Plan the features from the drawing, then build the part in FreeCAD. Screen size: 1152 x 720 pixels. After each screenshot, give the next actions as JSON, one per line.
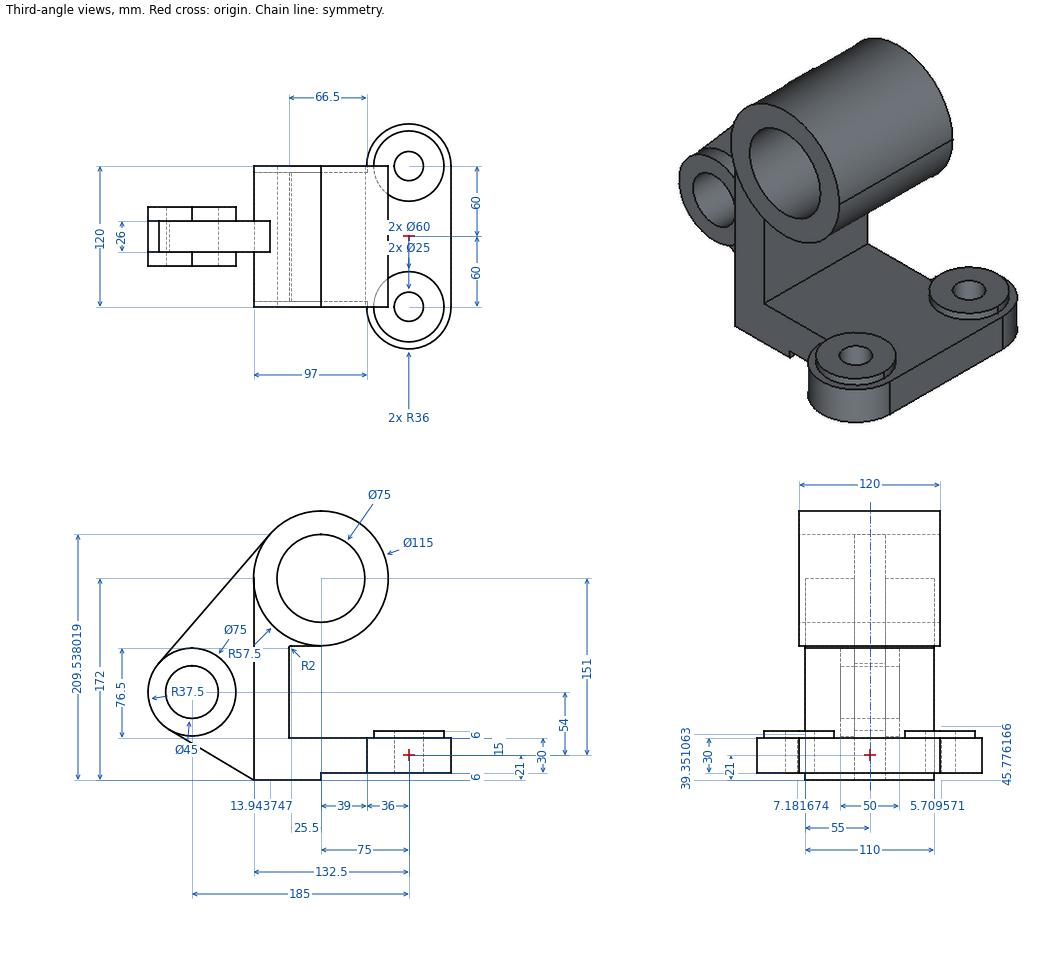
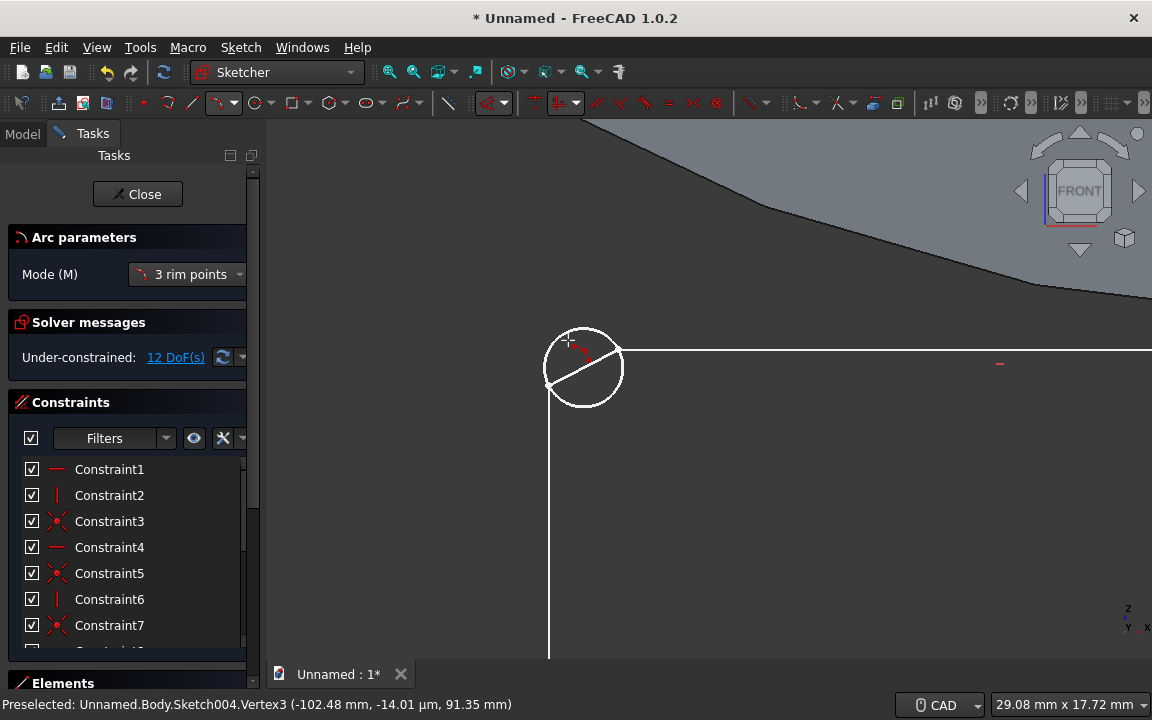
{"action": "left_click", "coordinate": [566, 338]}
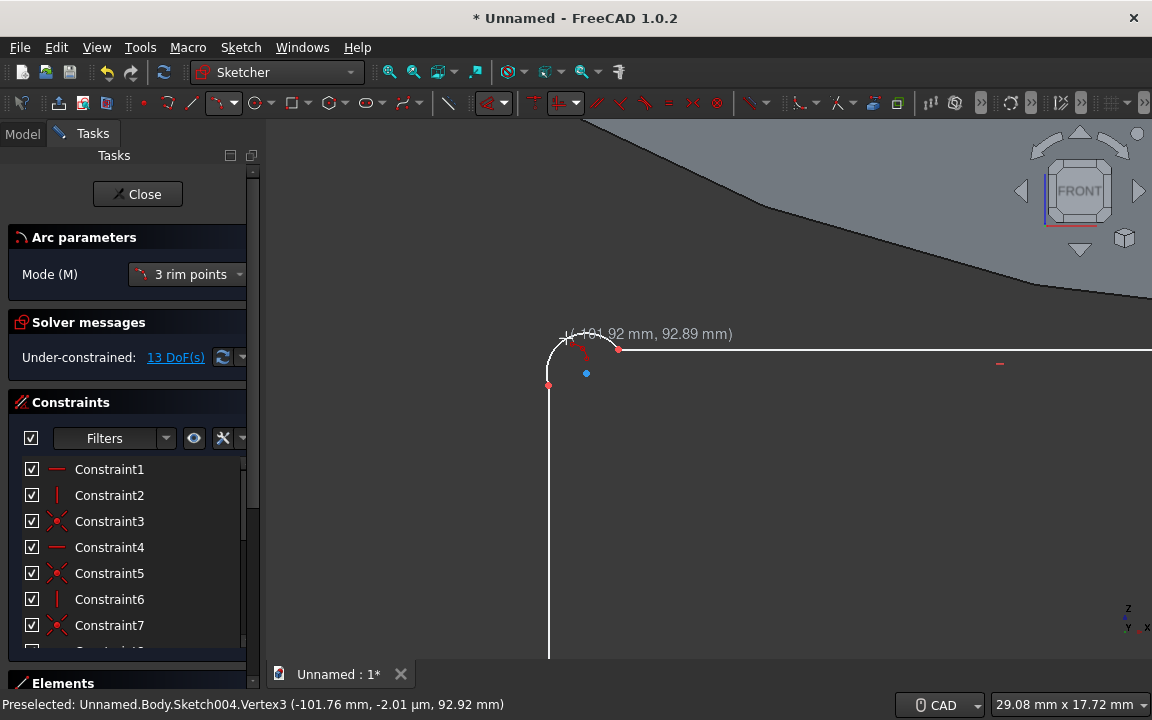
{"action": "scroll", "coordinate": [575, 337], "scroll_direction": "down", "scroll_amount": 14}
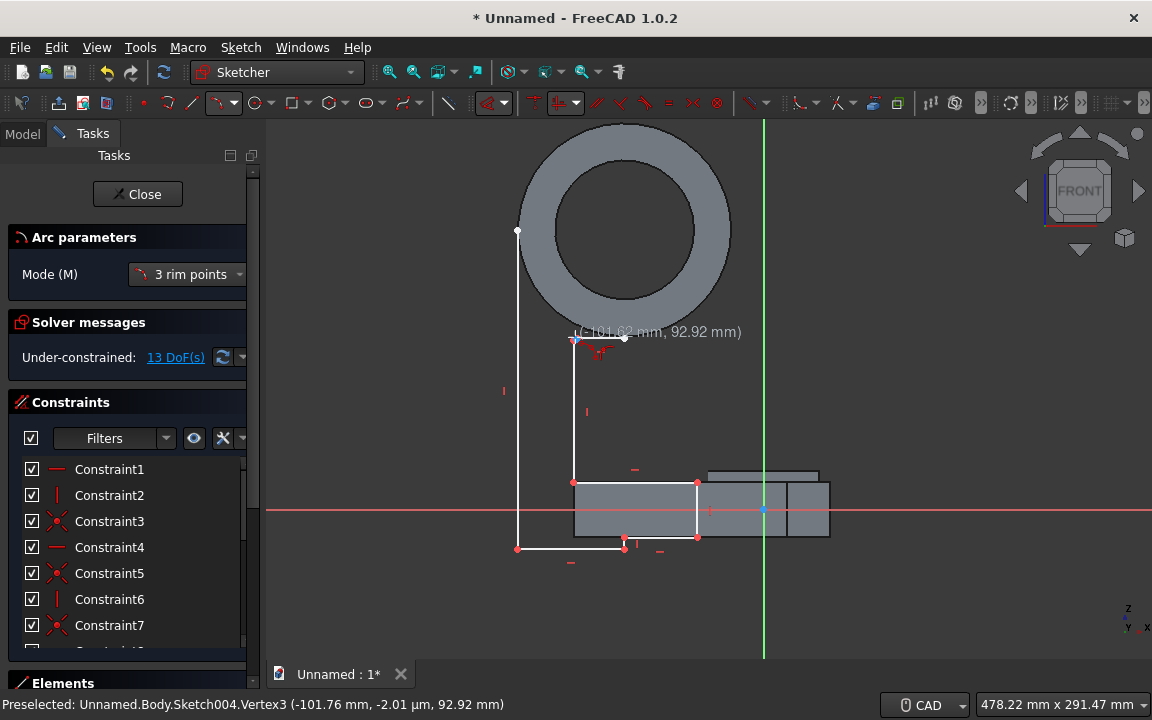
{"action": "left_click", "coordinate": [518, 231]}
{"action": "left_click", "coordinate": [624, 338]}
{"action": "left_click", "coordinate": [549, 305]}
{"action": "key", "text": "Escape"}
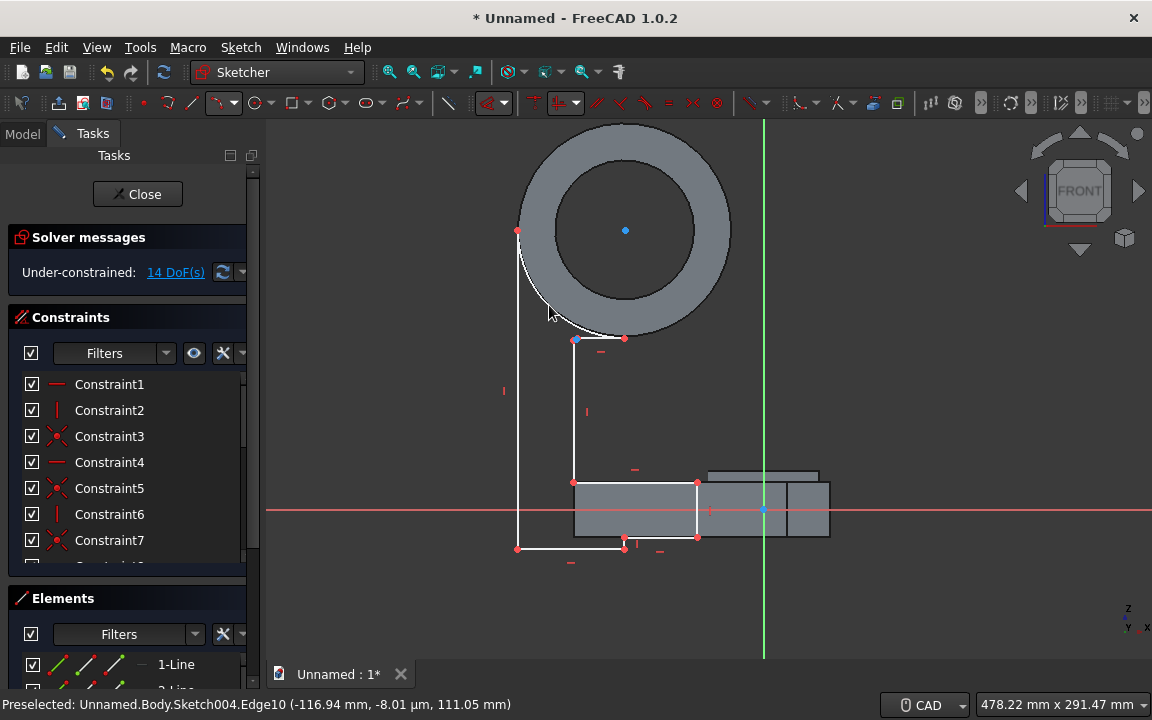
{"action": "scroll", "coordinate": [587, 338], "scroll_direction": "up", "scroll_amount": 4}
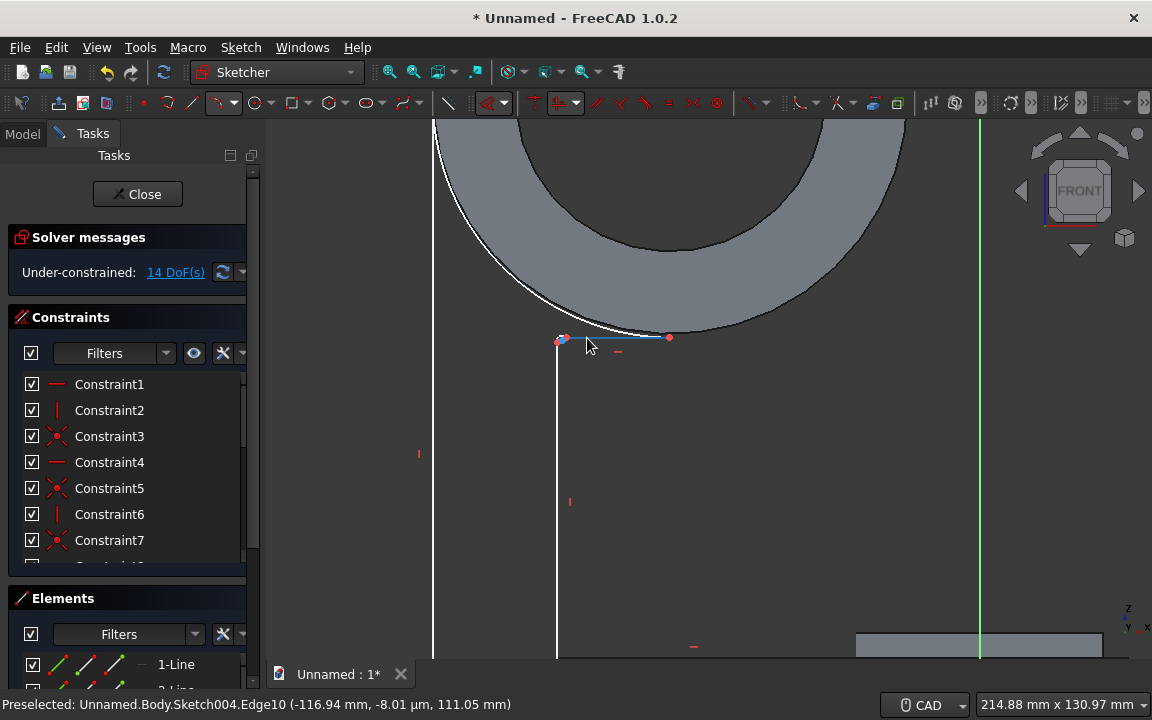
{"action": "left_click", "coordinate": [587, 338]}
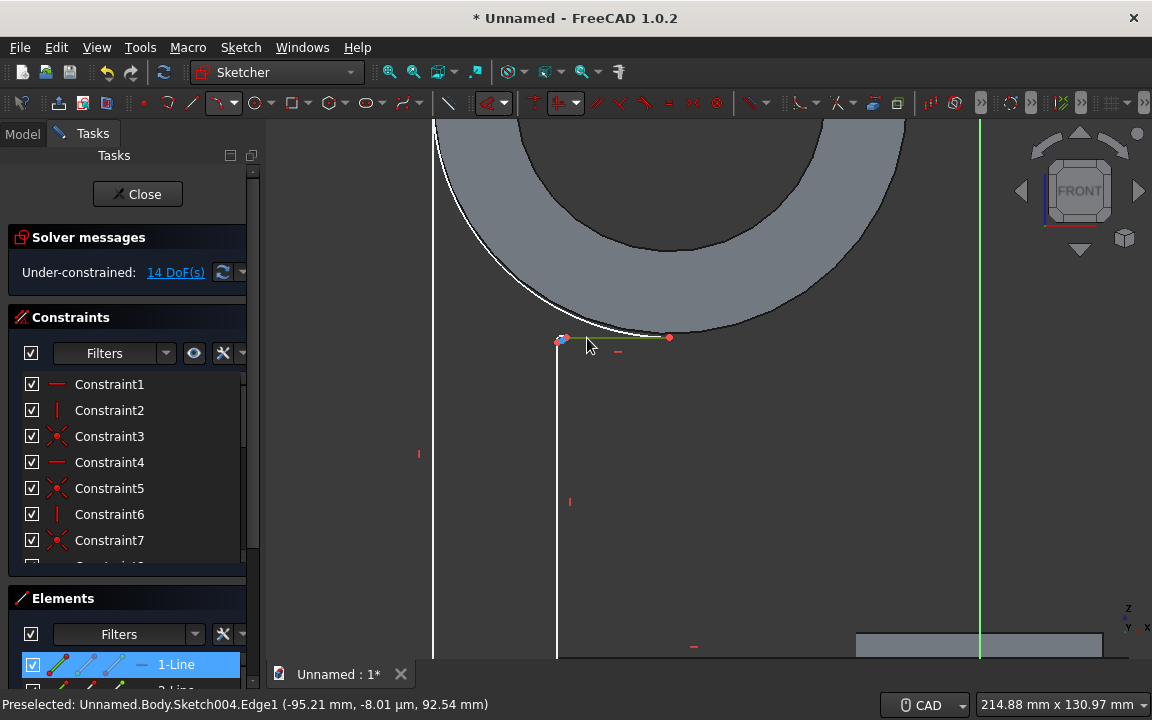
{"action": "scroll", "coordinate": [560, 336], "scroll_direction": "up", "scroll_amount": 5}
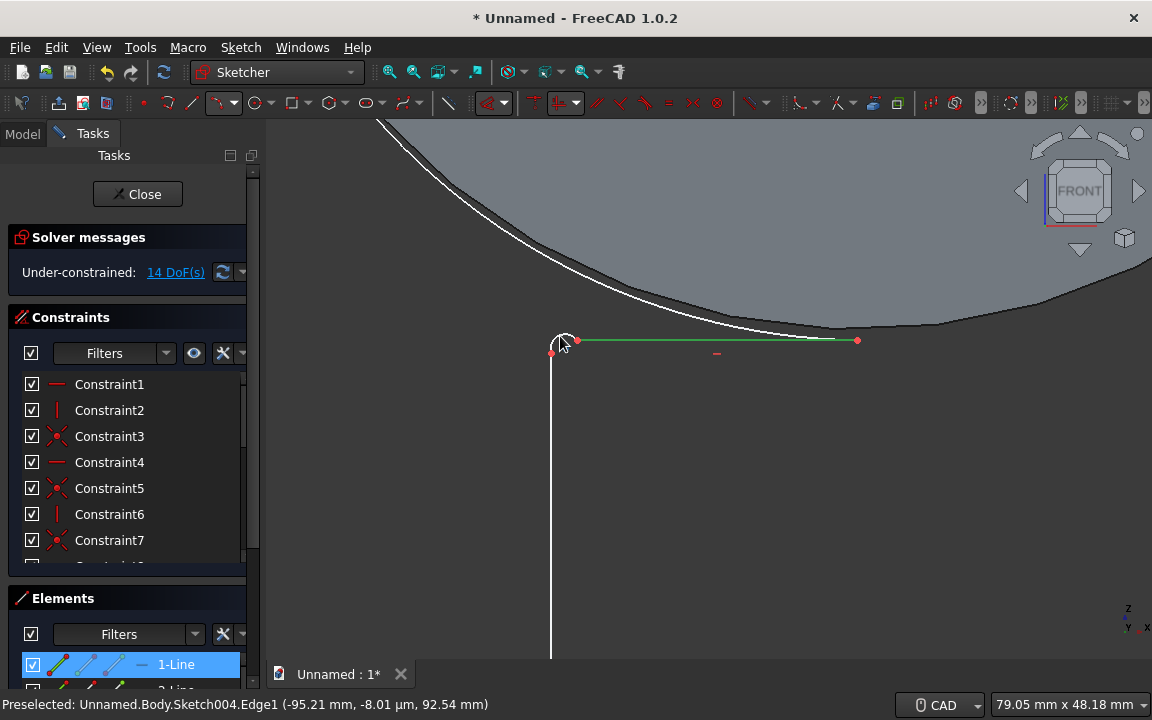
{"action": "left_click", "coordinate": [558, 336]}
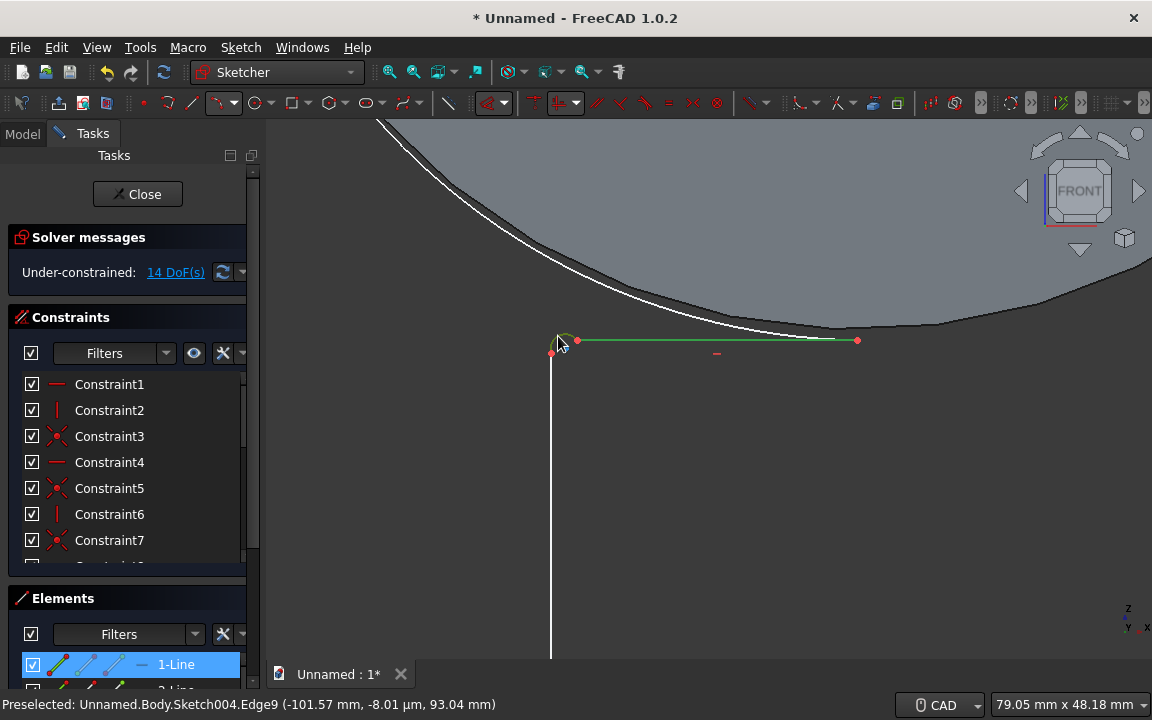
{"action": "key", "text": "t"}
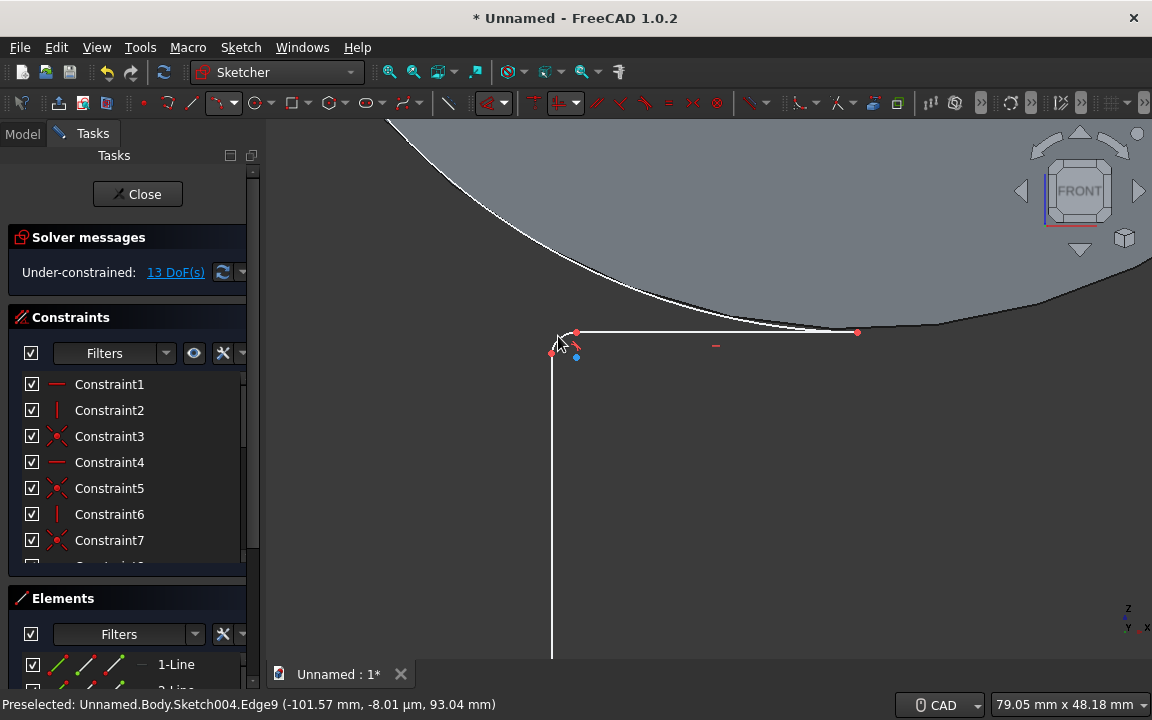
{"action": "scroll", "coordinate": [578, 338], "scroll_direction": "down", "scroll_amount": 9}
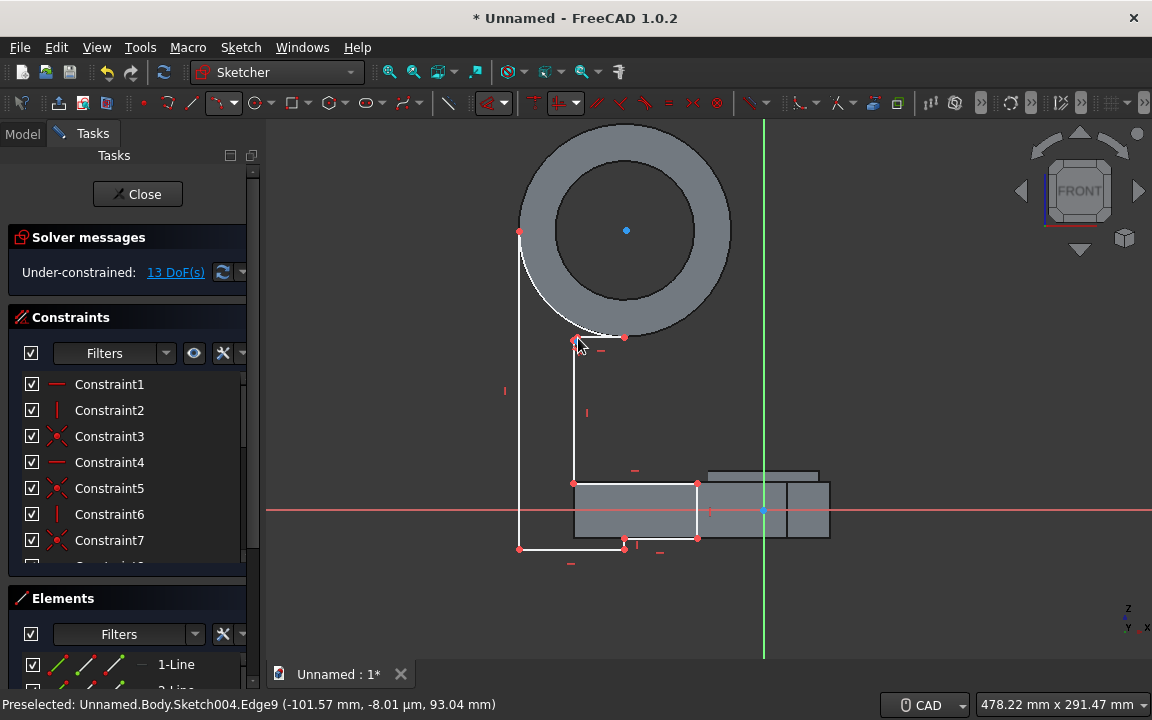
{"action": "left_click", "coordinate": [574, 384]}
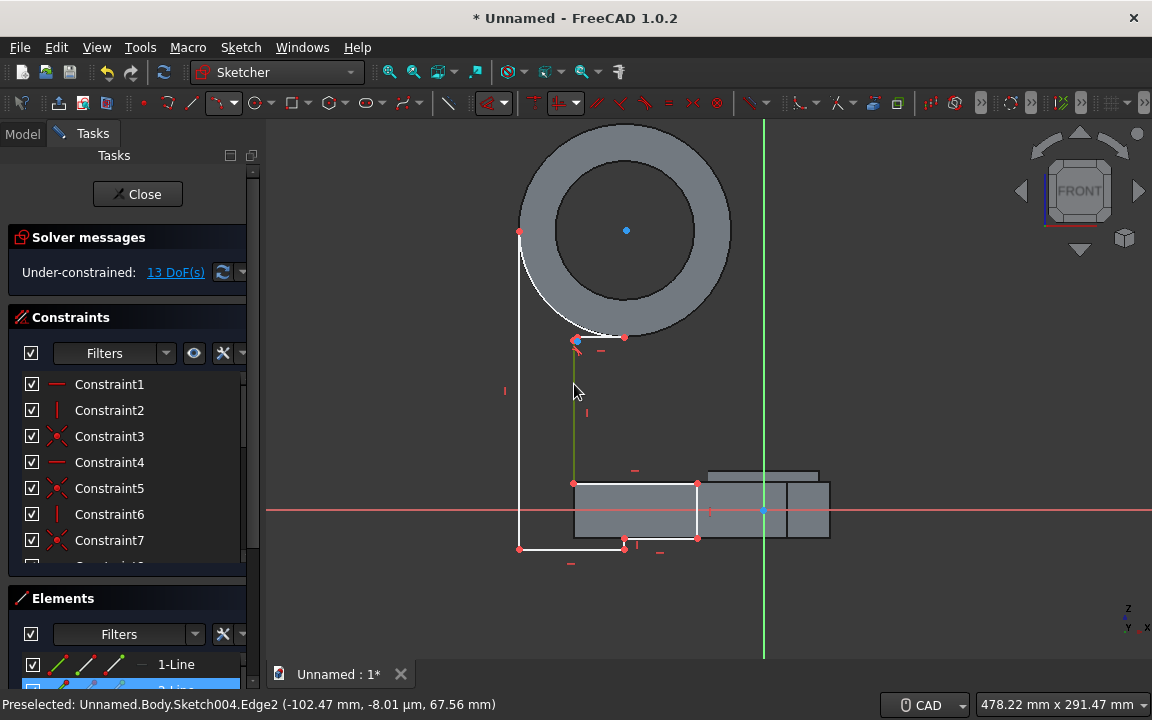
{"action": "scroll", "coordinate": [575, 338], "scroll_direction": "up", "scroll_amount": 8}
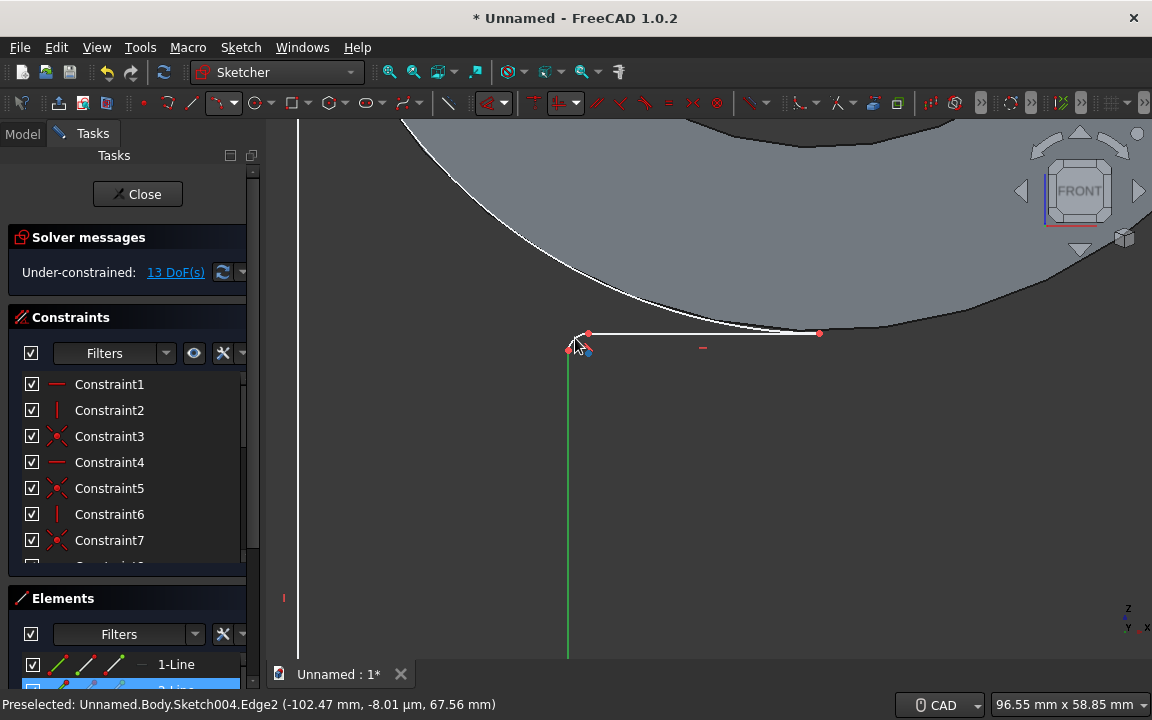
{"action": "left_click", "coordinate": [575, 338]}